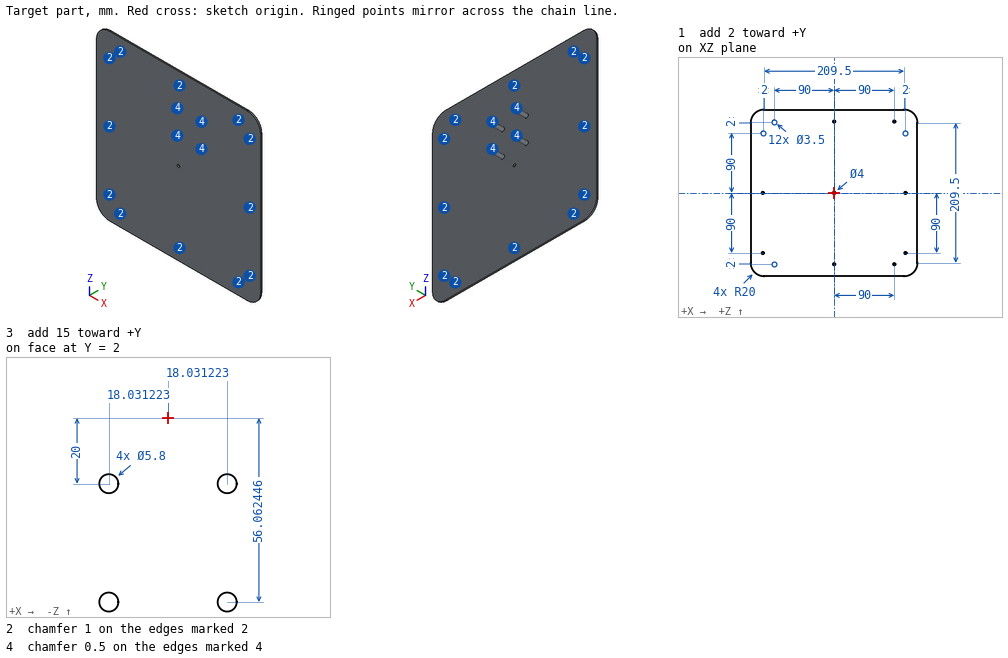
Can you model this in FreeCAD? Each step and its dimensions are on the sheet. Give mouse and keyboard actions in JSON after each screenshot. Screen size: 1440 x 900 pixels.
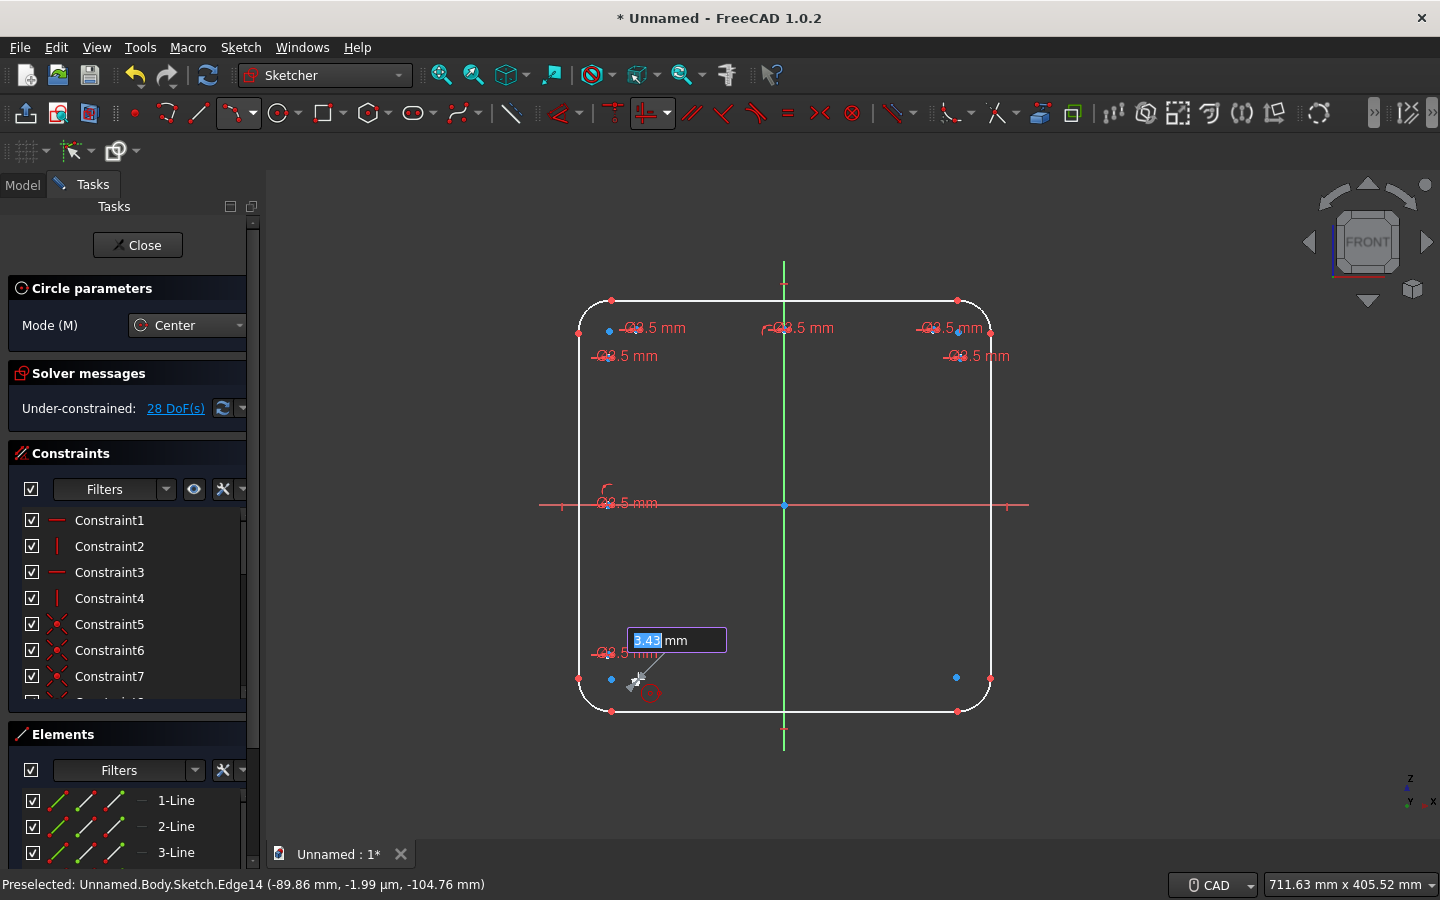
{"action": "type", "text": "3.5"}
{"action": "key", "text": "Return"}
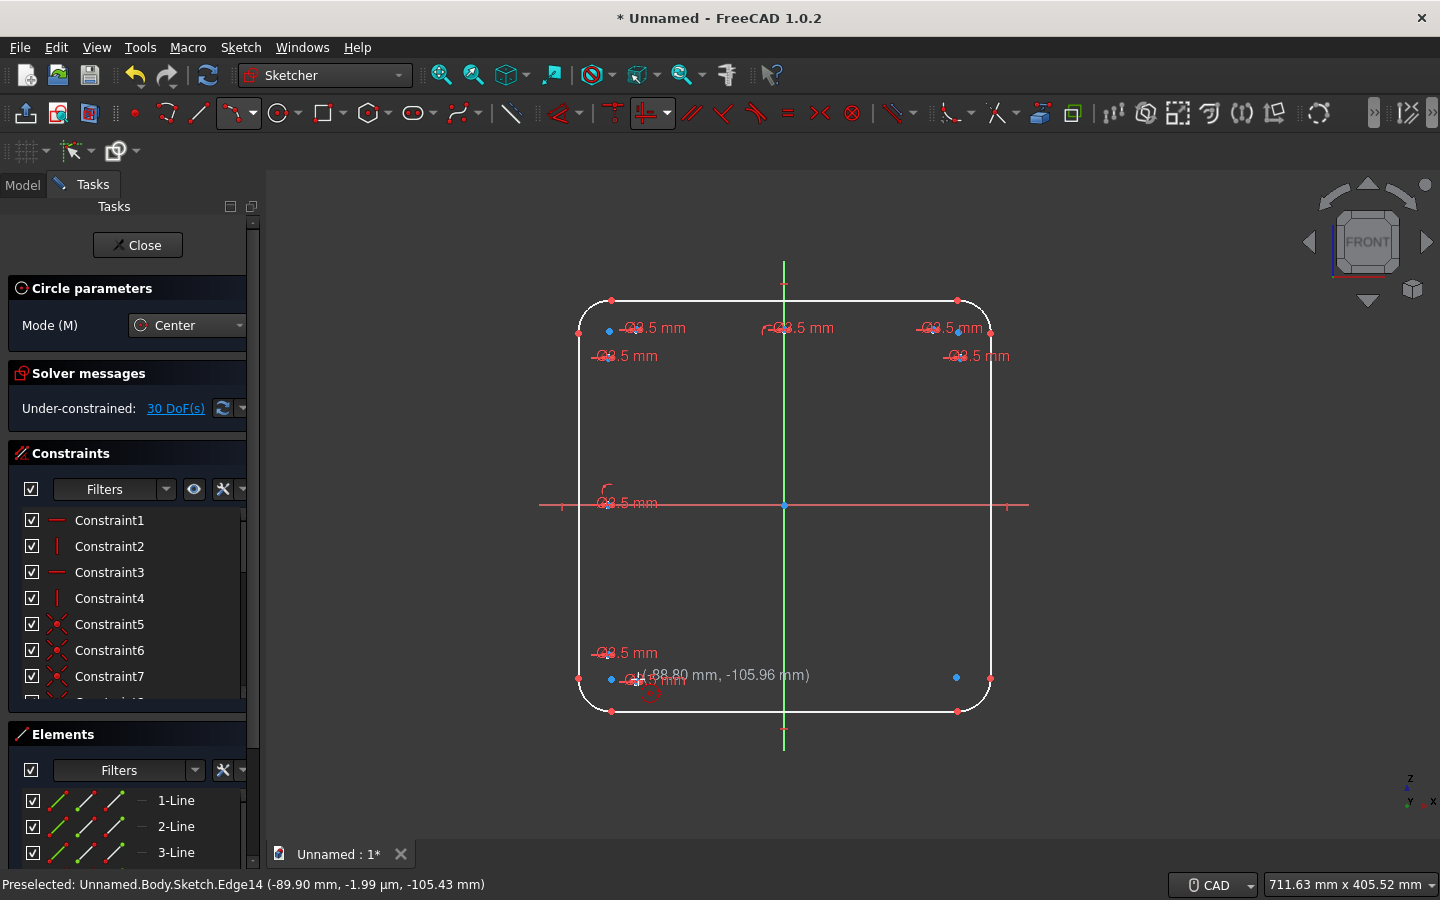
{"action": "scroll", "coordinate": [784, 505], "scroll_direction": "up", "scroll_amount": 10}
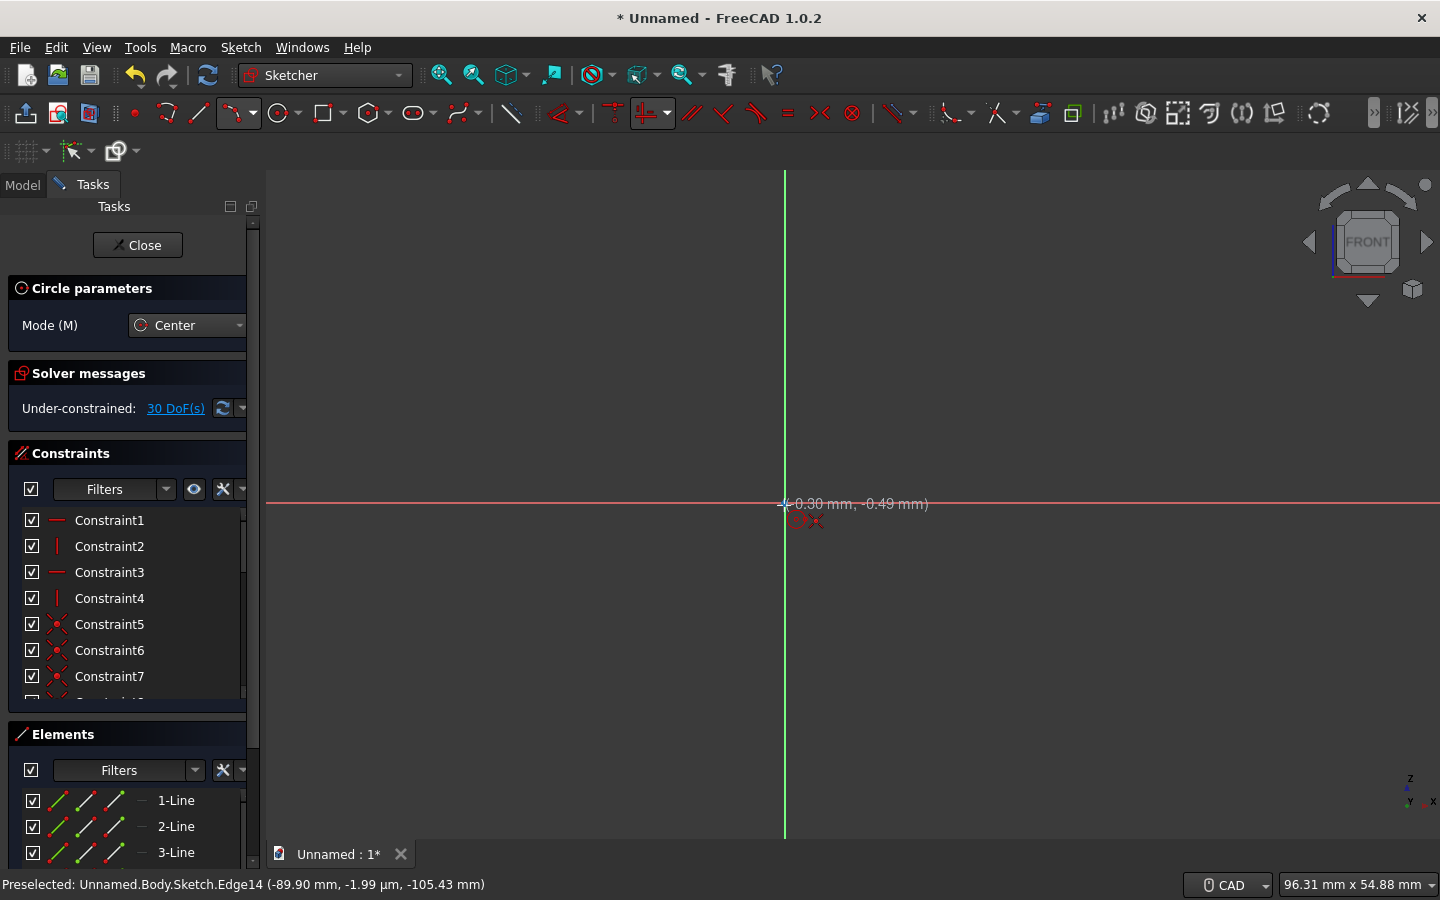
{"action": "scroll", "coordinate": [784, 505], "scroll_direction": "down", "scroll_amount": 10}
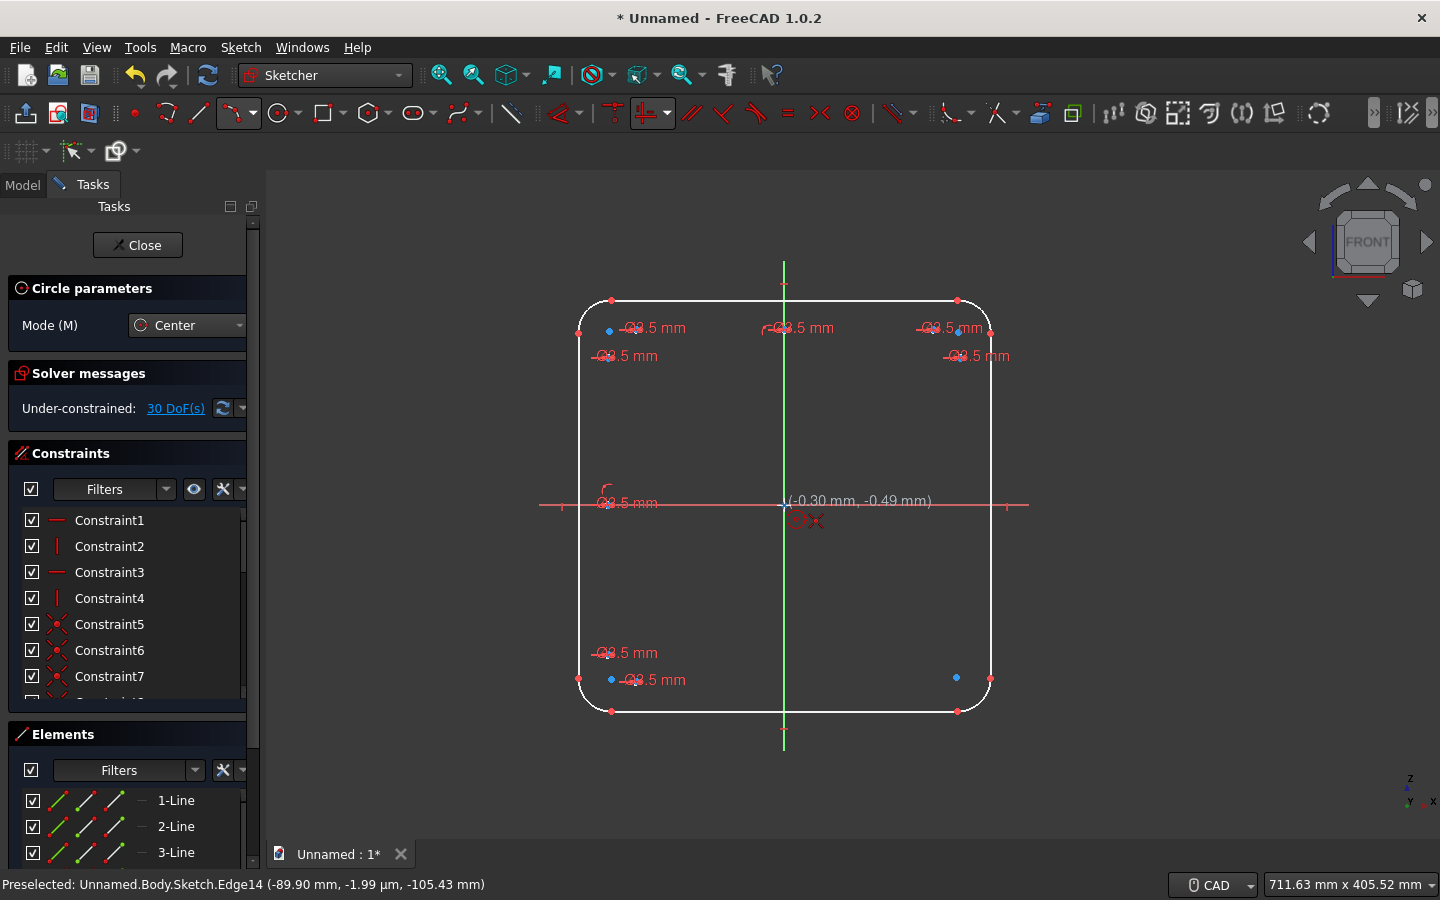
{"action": "left_click", "coordinate": [784, 505]}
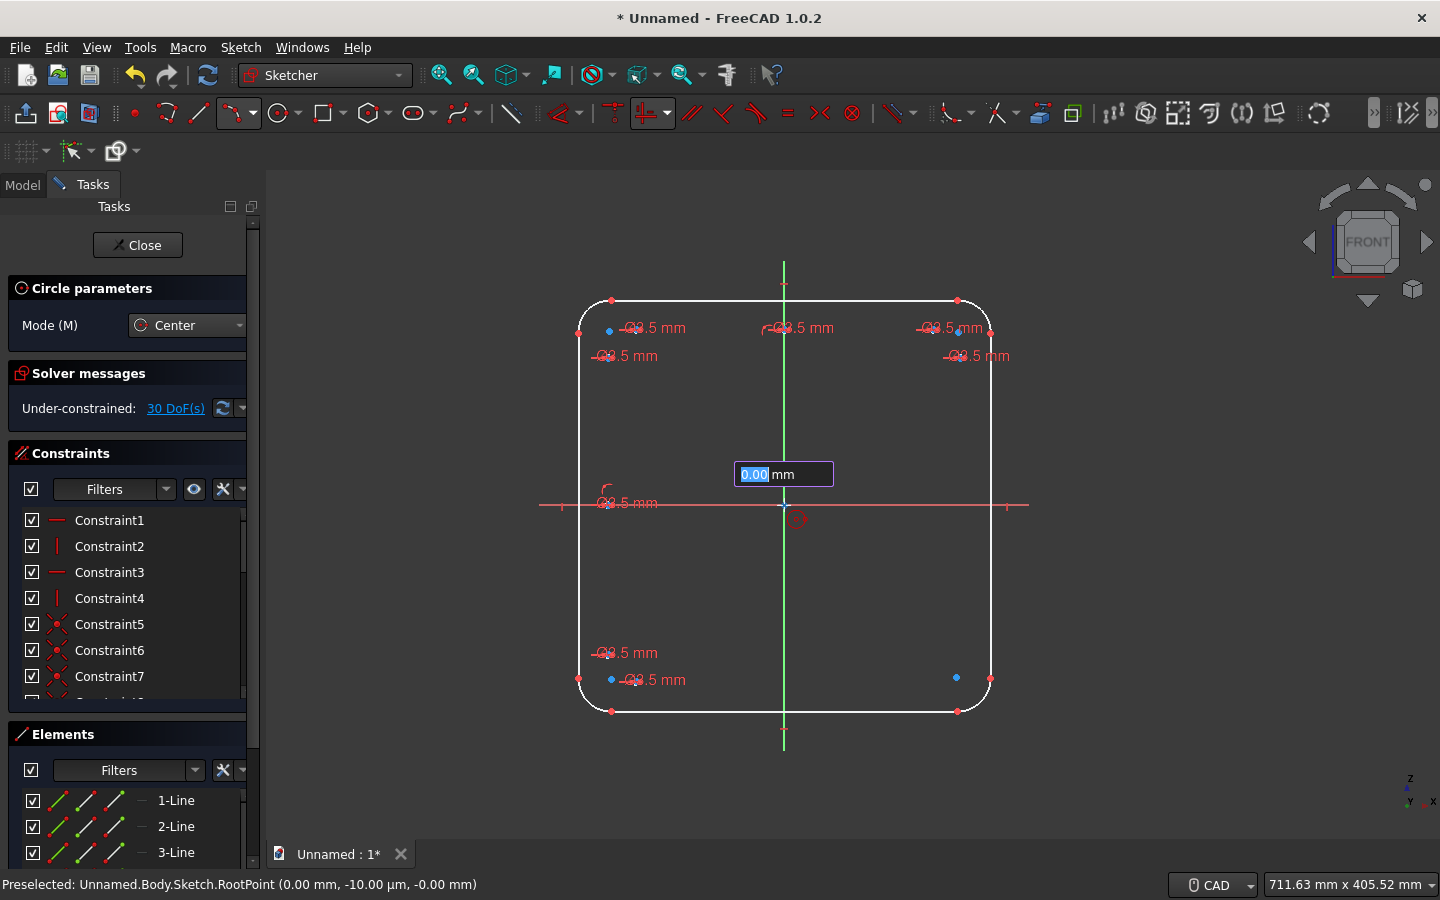
{"action": "scroll", "coordinate": [787, 503], "scroll_direction": "up", "scroll_amount": 10}
{"action": "mouse_move", "coordinate": [783, 499]}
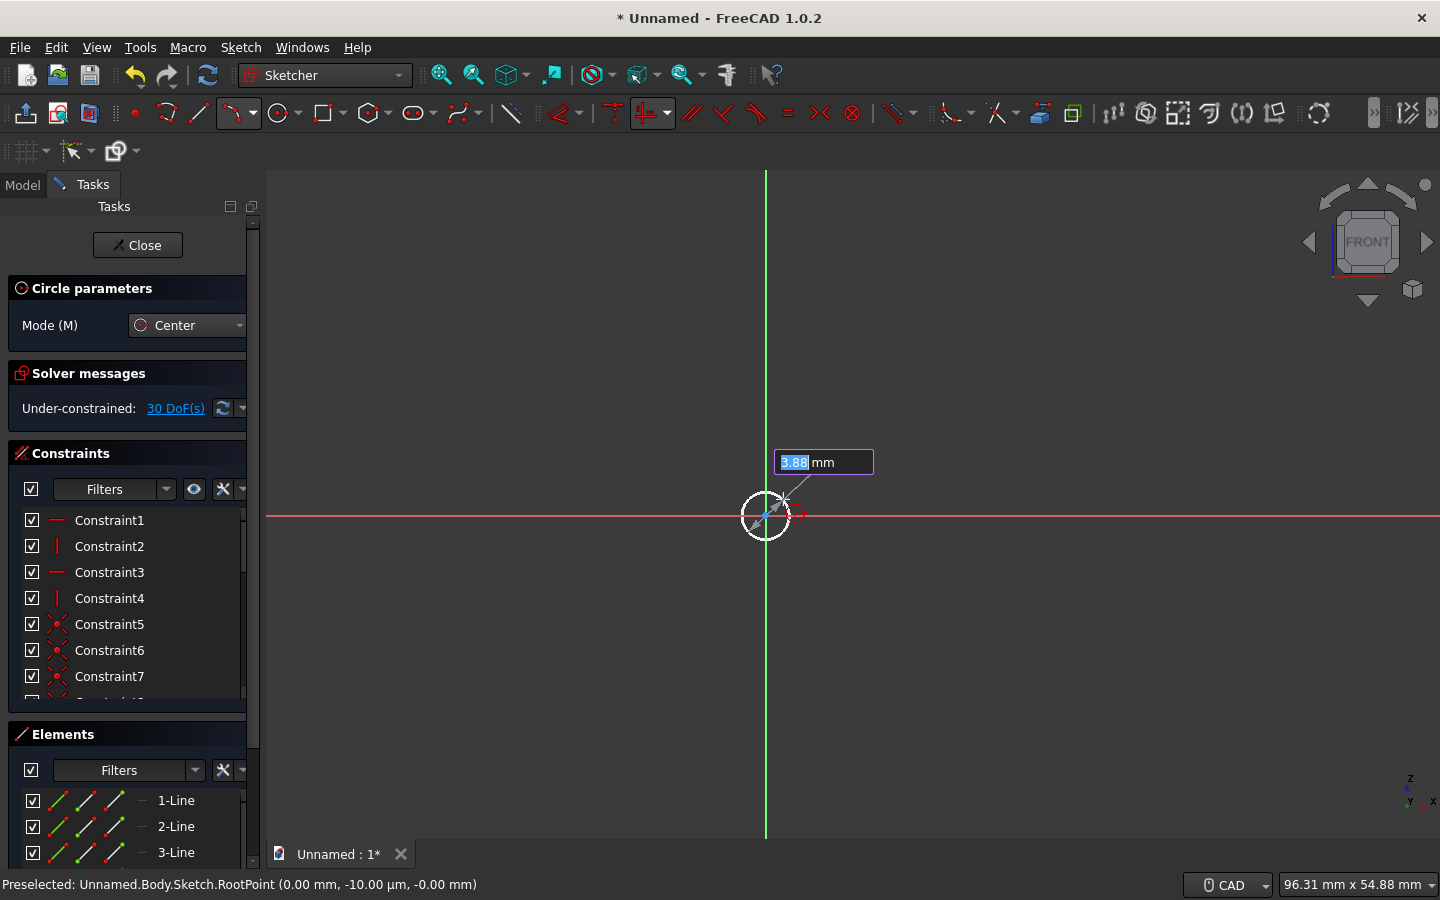
{"action": "type", "text": "4"}
{"action": "key", "text": "Return"}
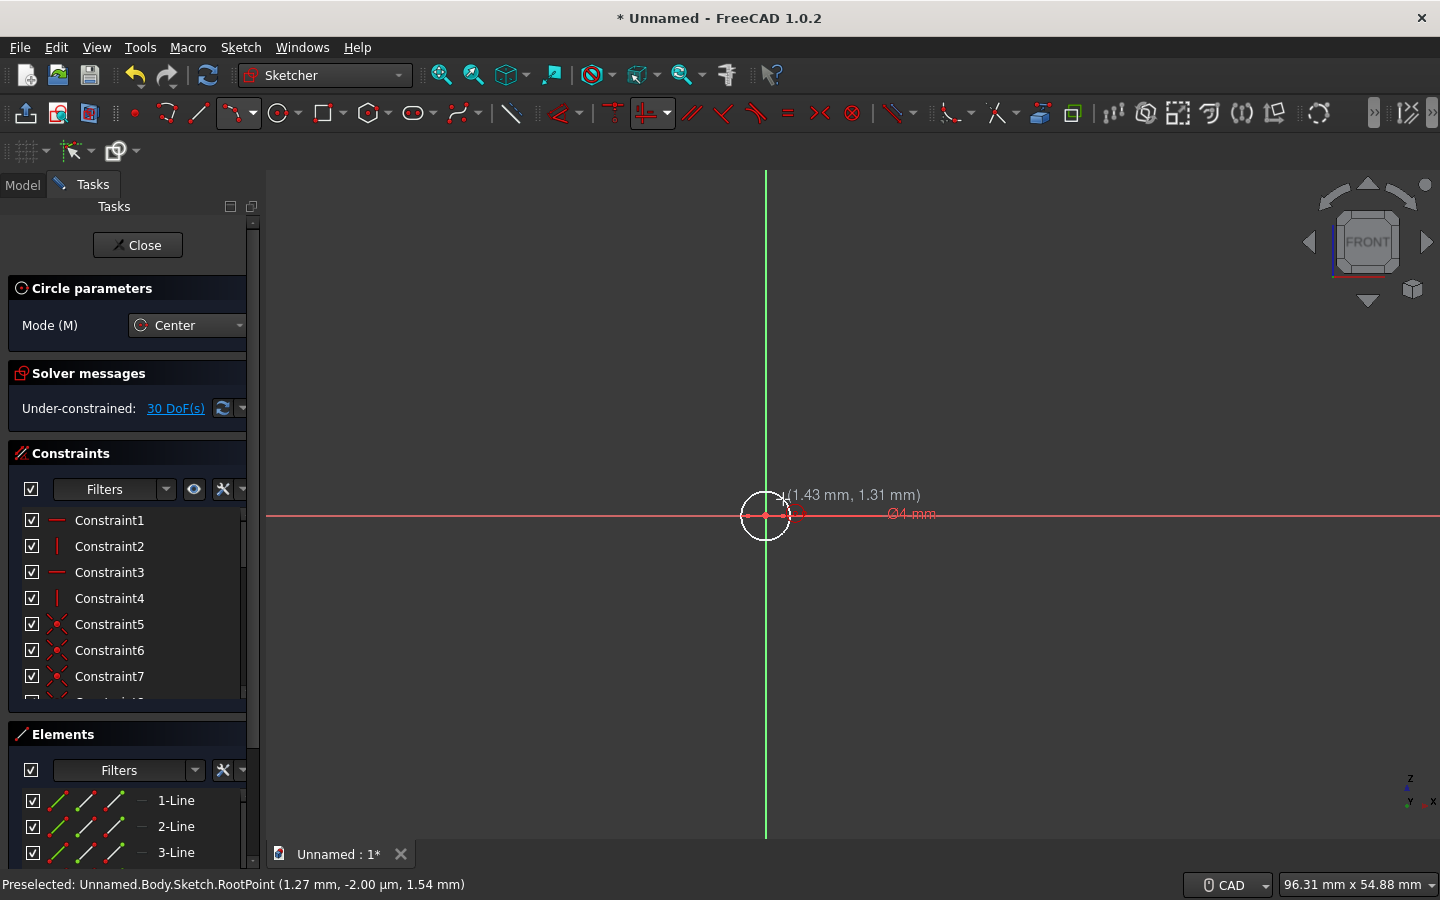
{"action": "scroll", "coordinate": [787, 503], "scroll_direction": "down", "scroll_amount": 10}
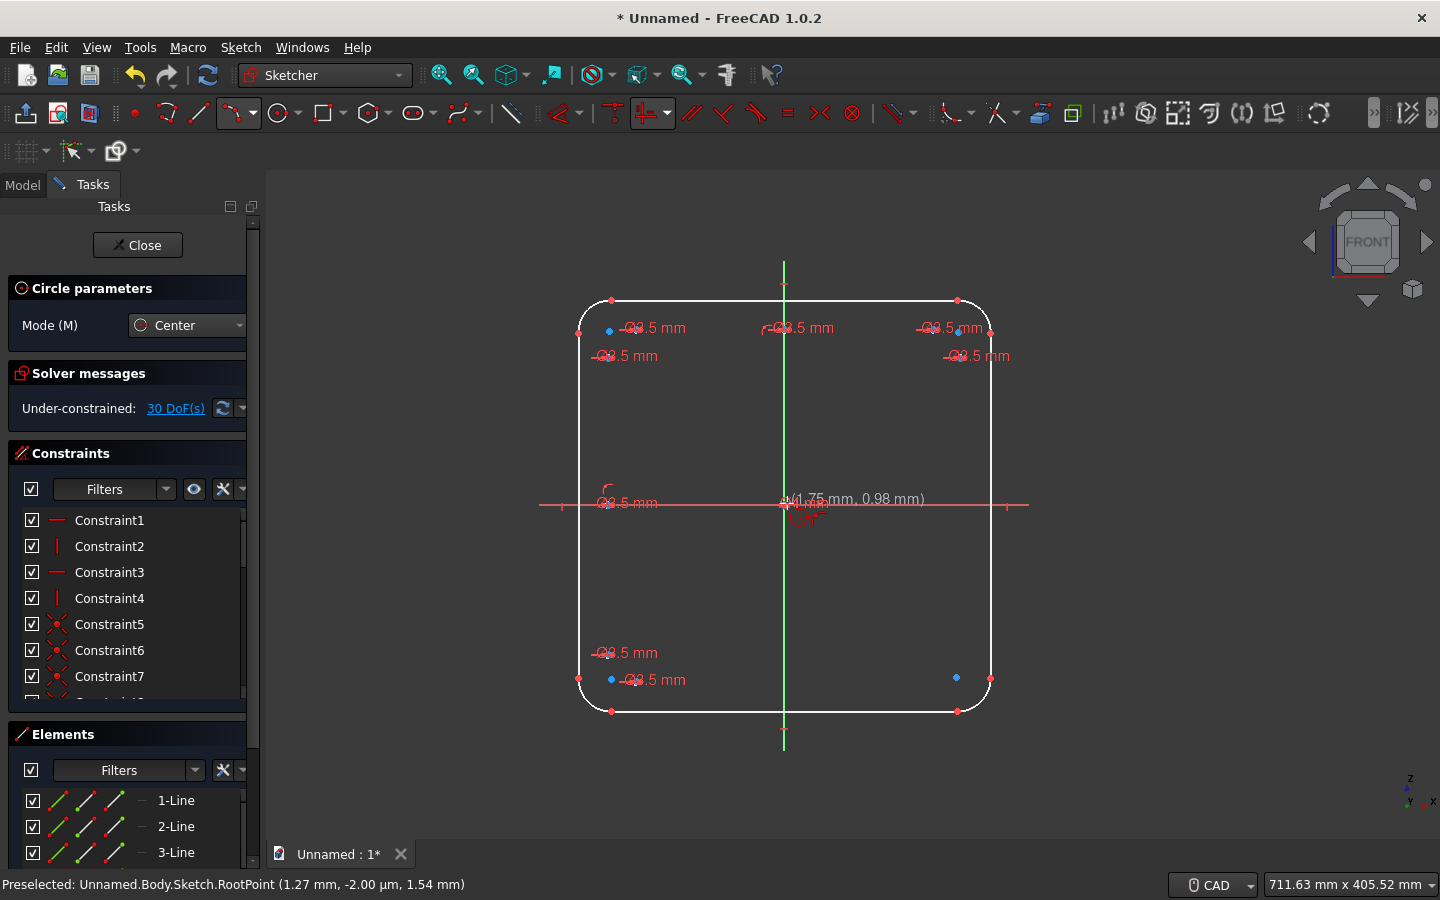
{"action": "scroll", "coordinate": [961, 505], "scroll_direction": "up", "scroll_amount": 11}